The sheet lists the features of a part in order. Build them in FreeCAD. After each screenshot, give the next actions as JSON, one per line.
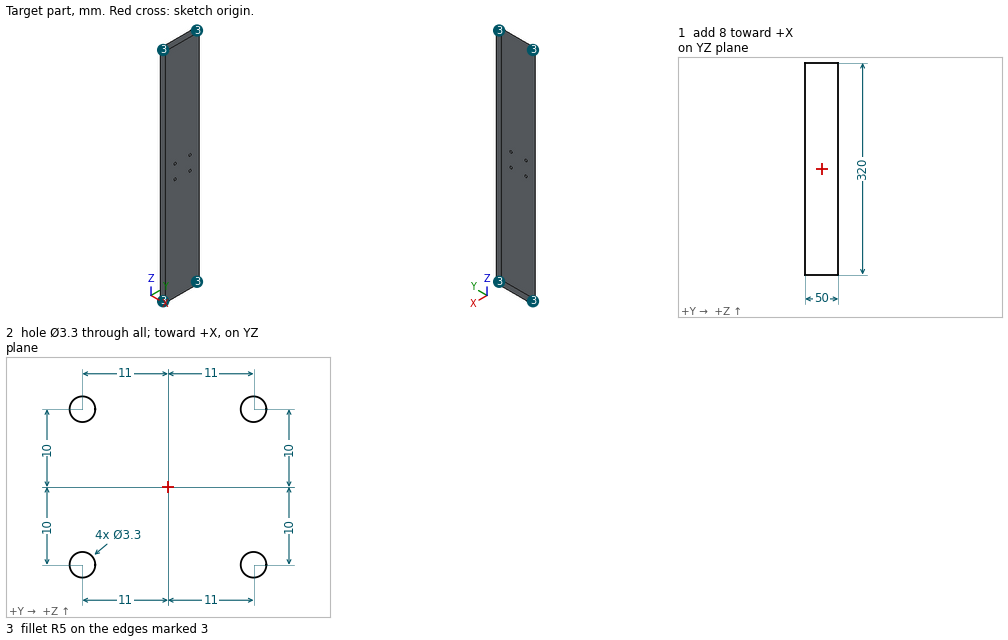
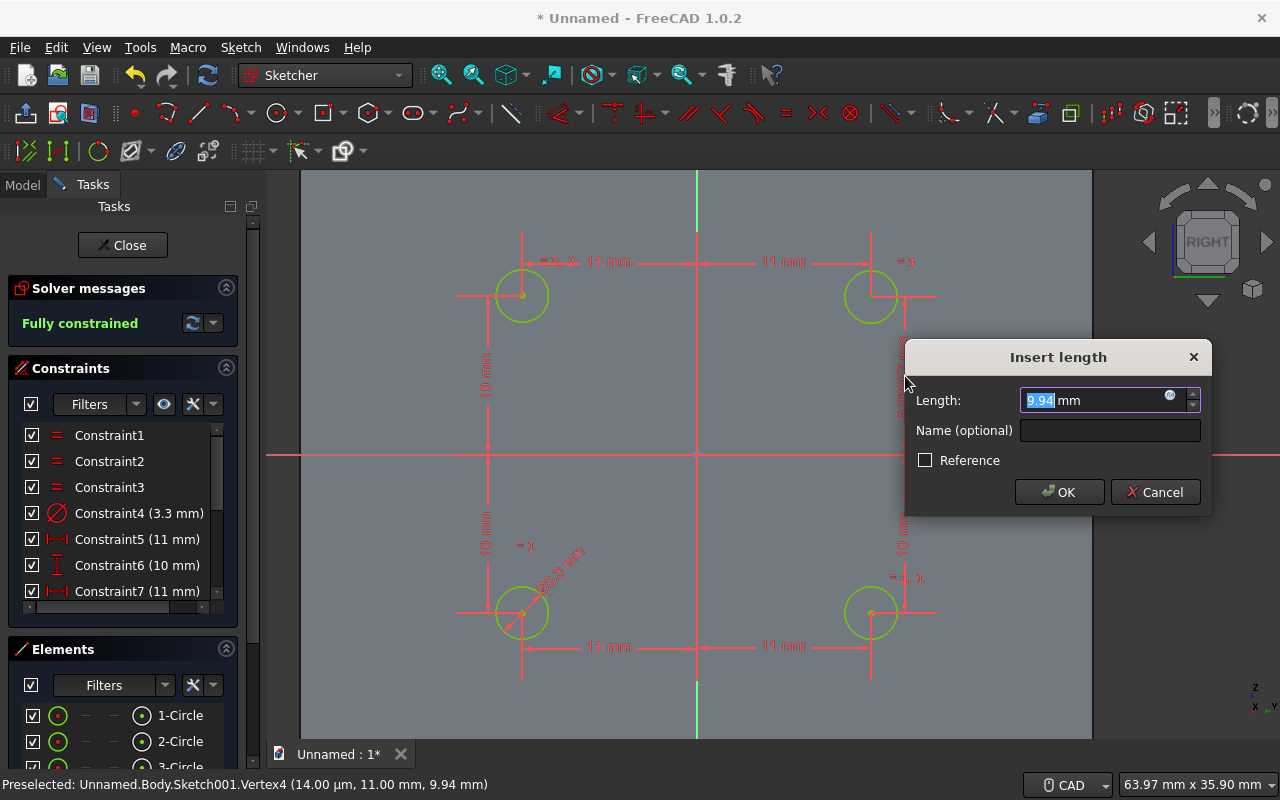
{"action": "type", "text": "10"}
{"action": "key", "text": "Return"}
{"action": "key", "text": "Escape"}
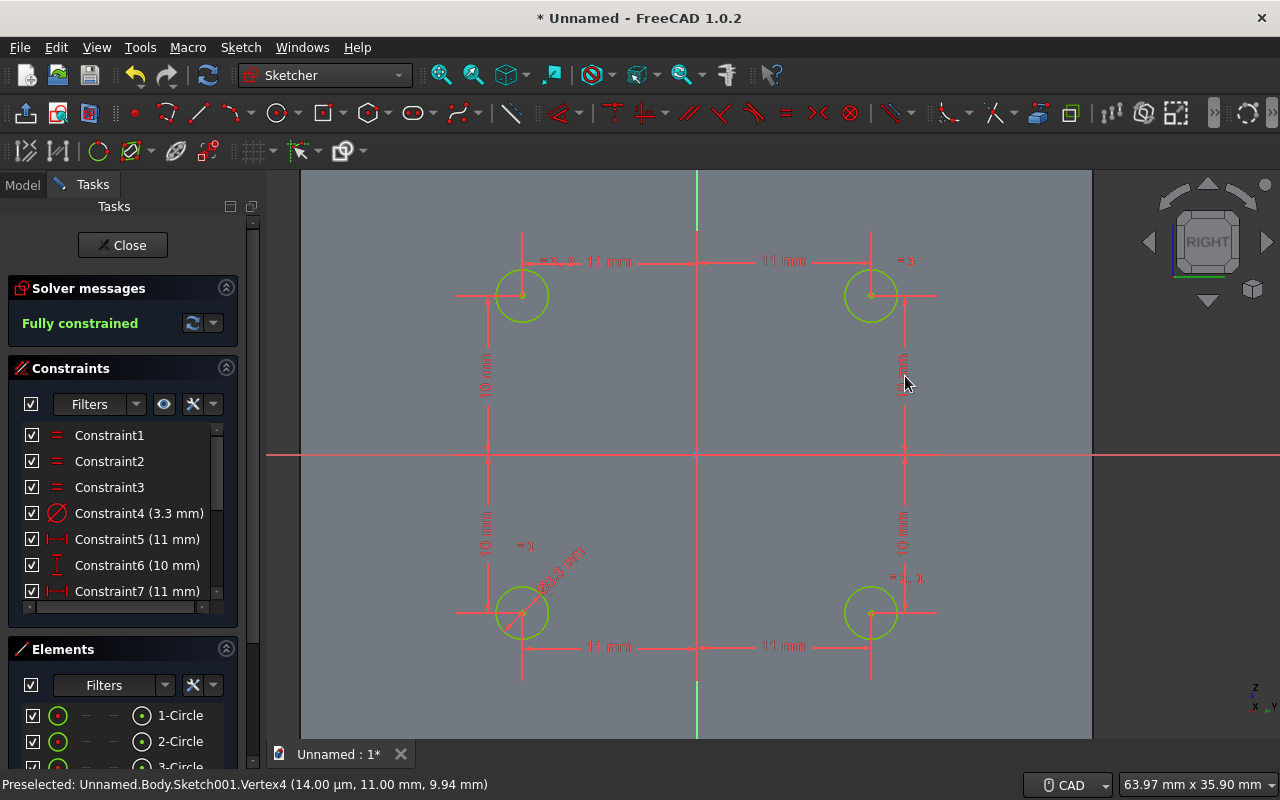
{"action": "left_click", "coordinate": [123, 245]}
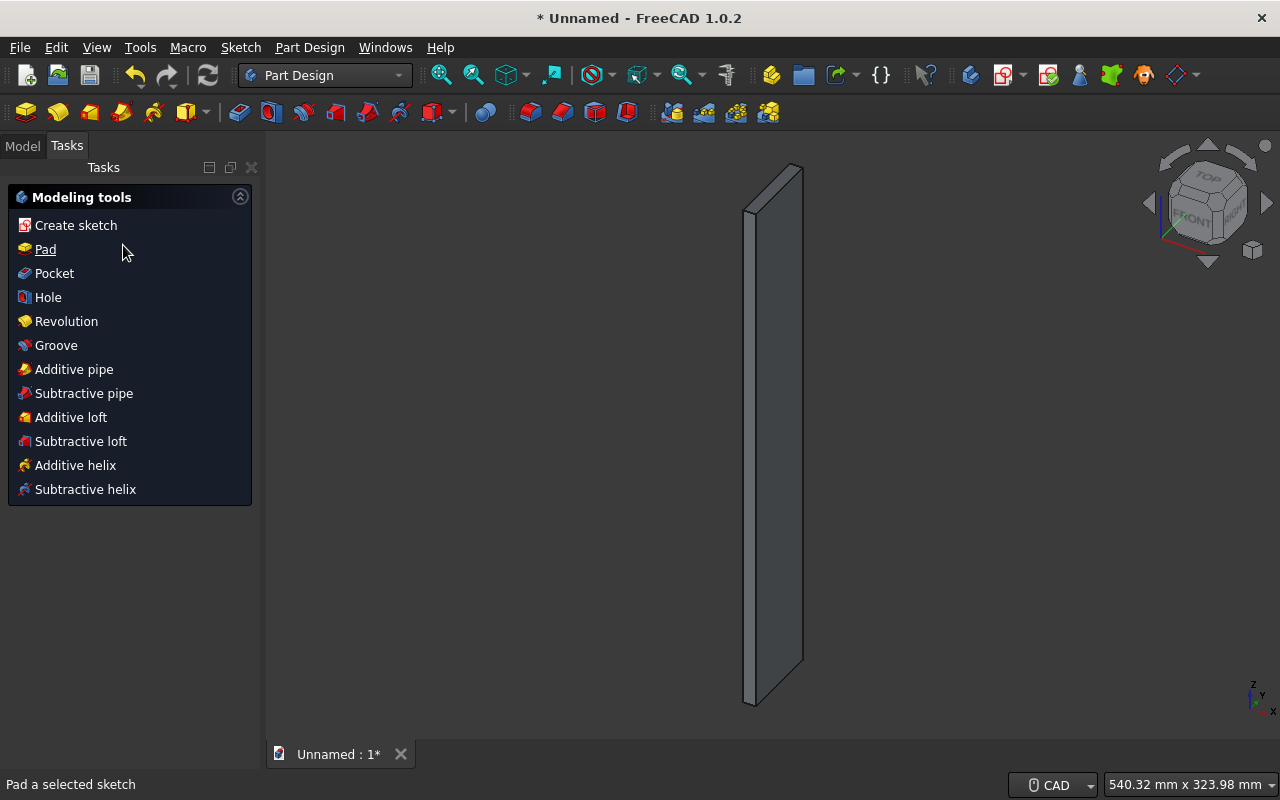
{"action": "left_click", "coordinate": [272, 112]}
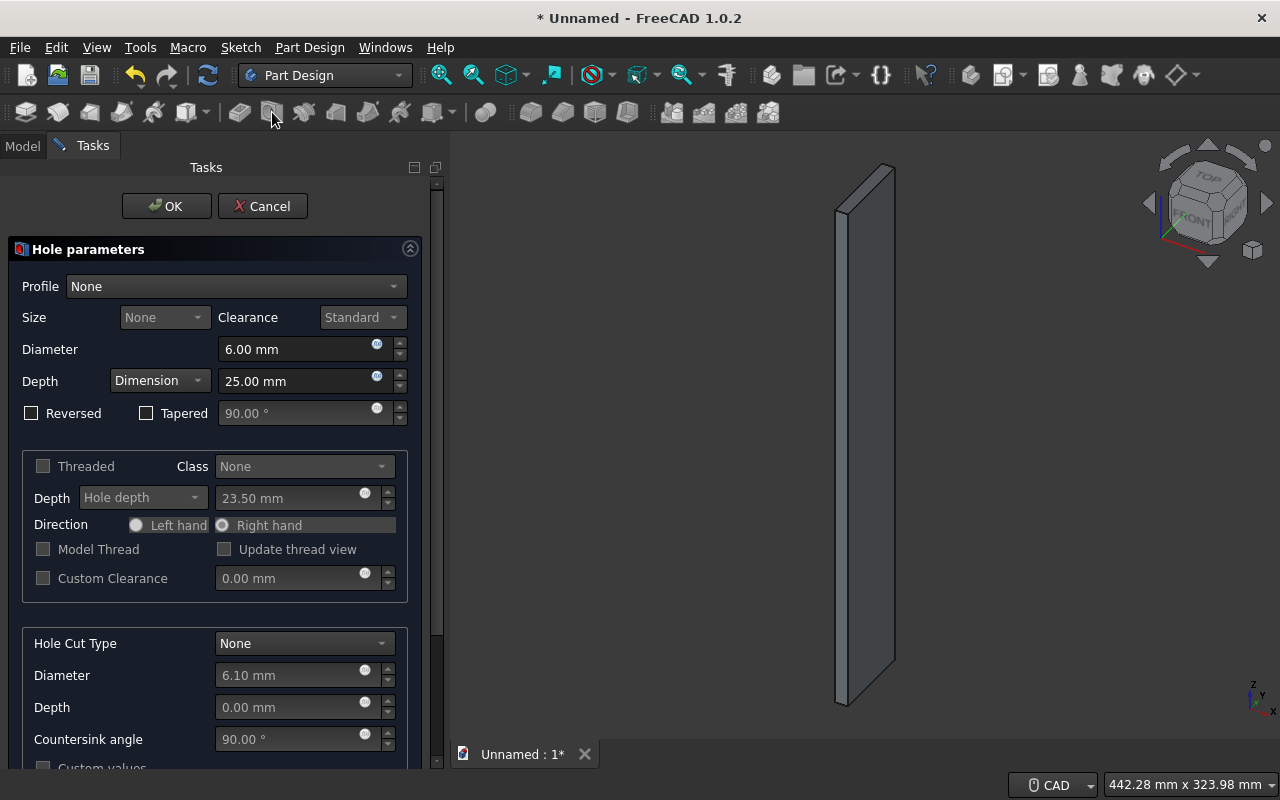
{"action": "triple_click", "coordinate": [305, 349]}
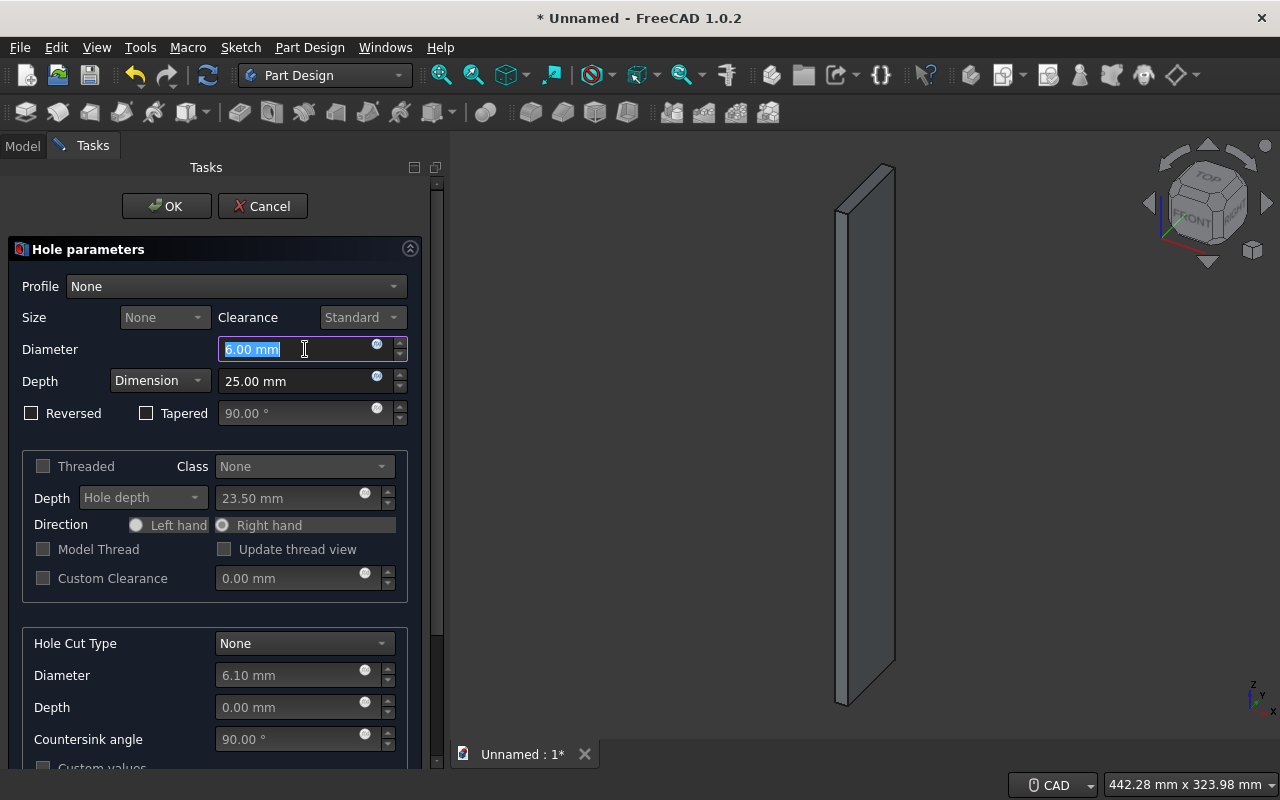
{"action": "type", "text": "3.3"}
{"action": "key", "text": "Tab"}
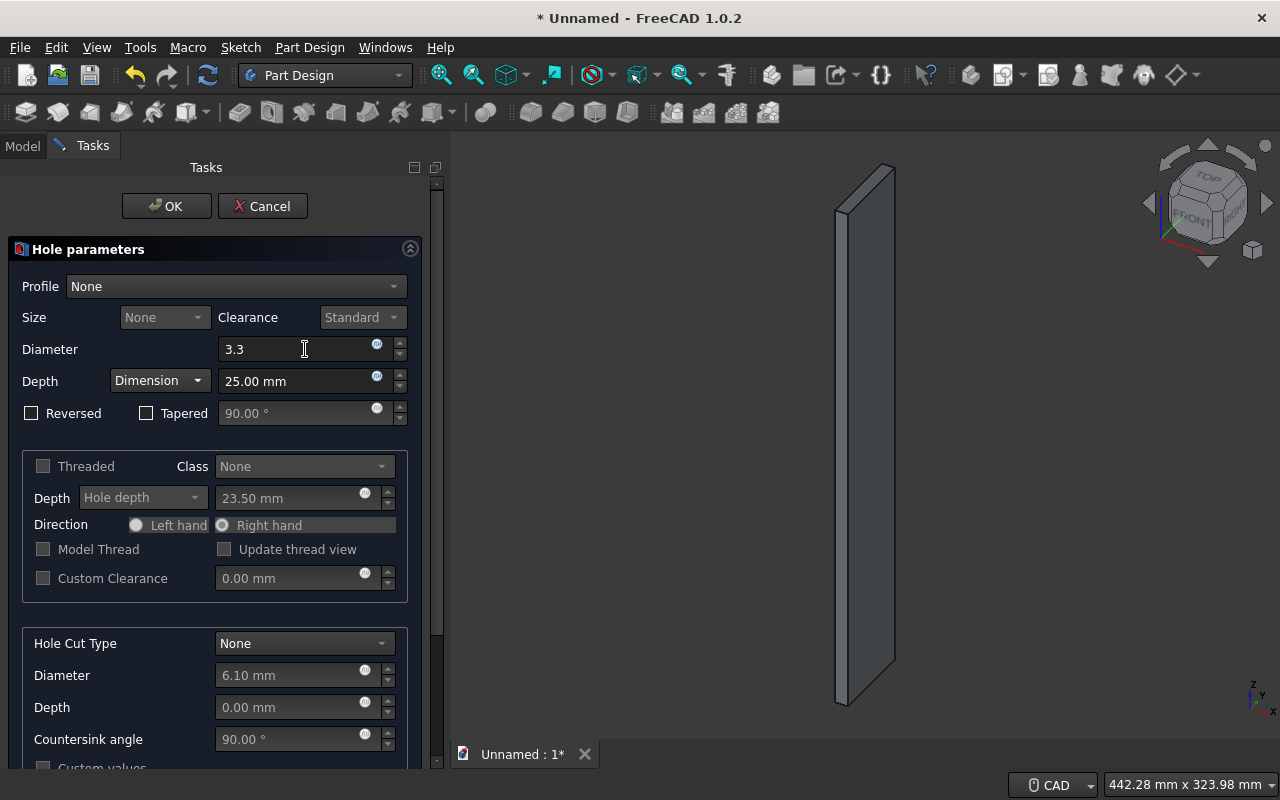
{"action": "left_click", "coordinate": [161, 380]}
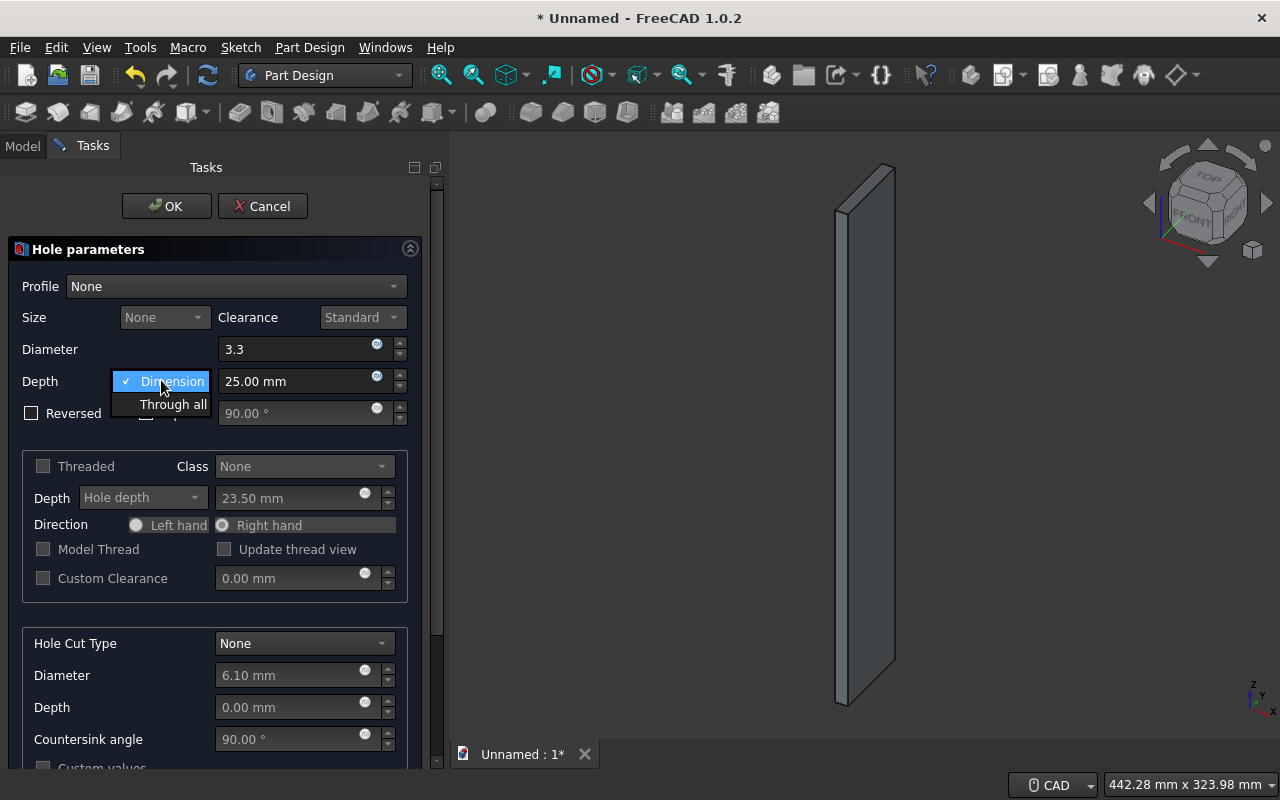
{"action": "left_click", "coordinate": [160, 404]}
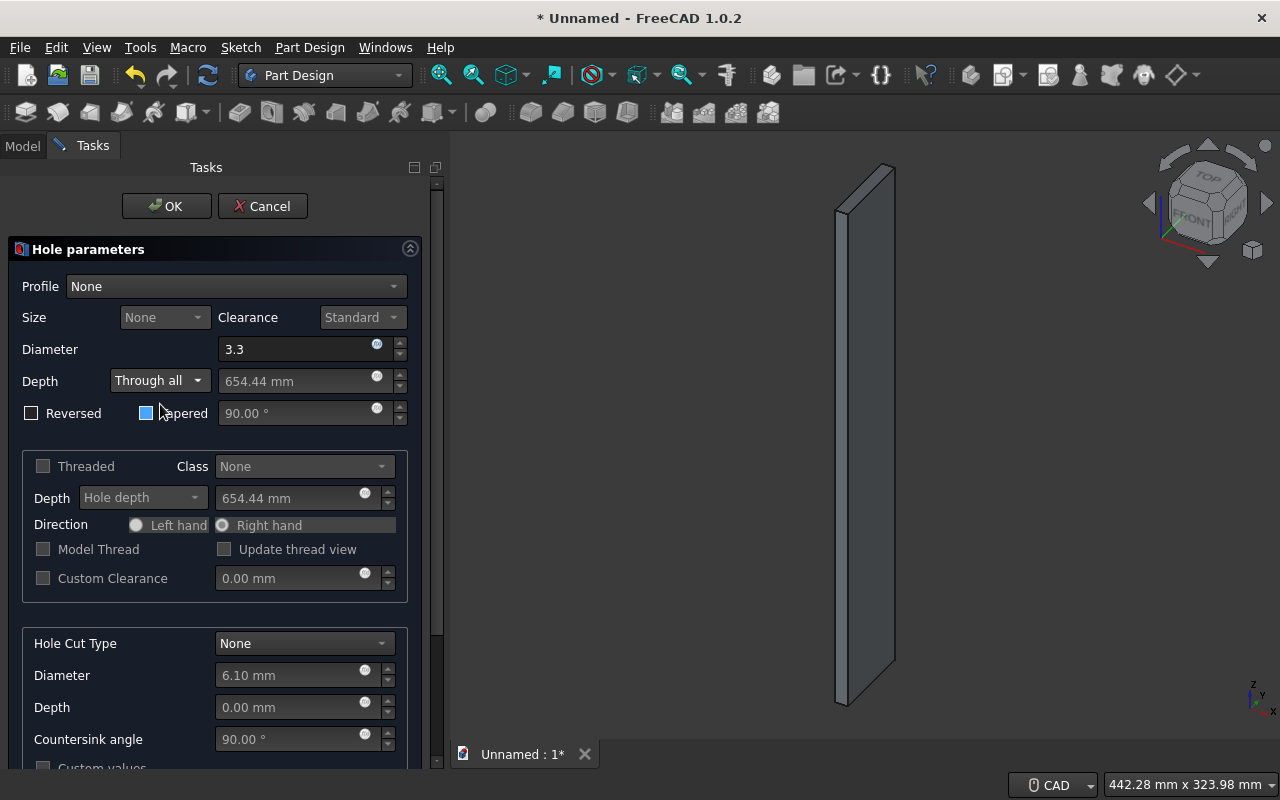
{"action": "left_click", "coordinate": [30, 413]}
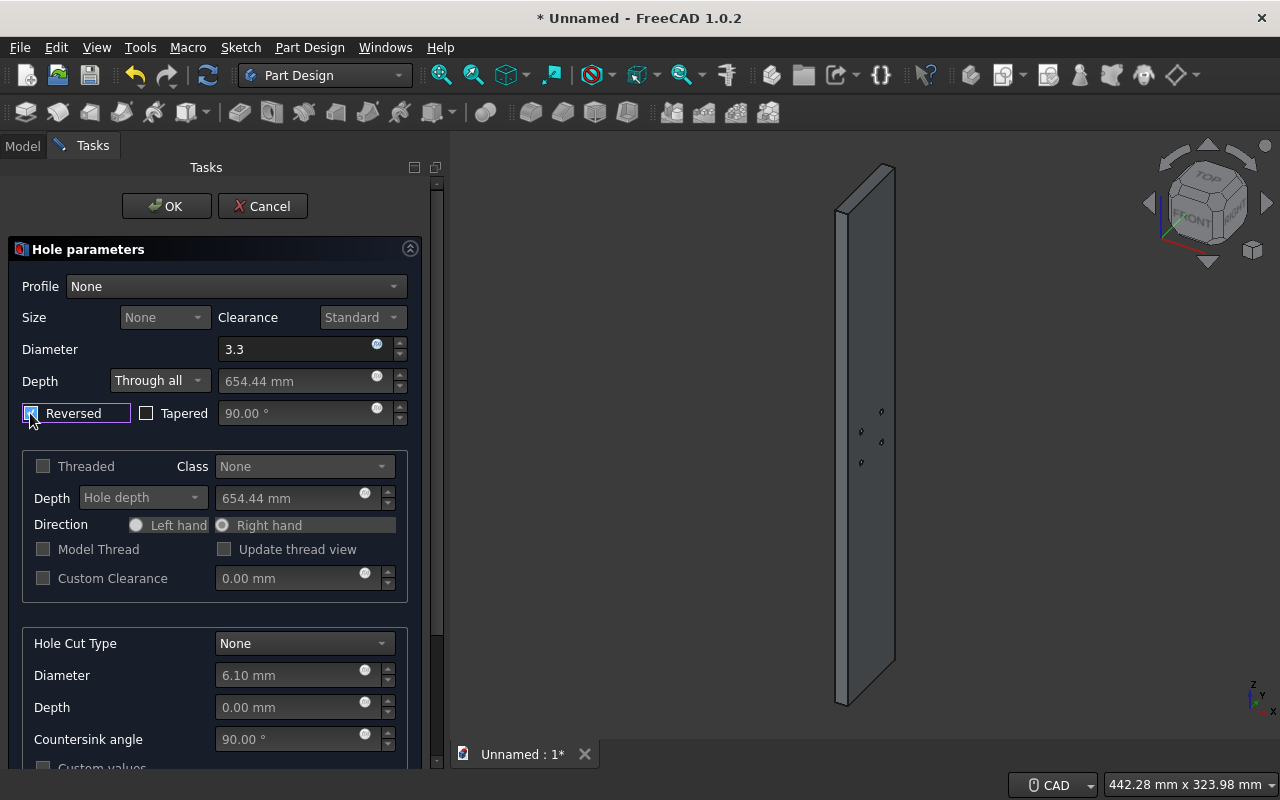
{"action": "left_click", "coordinate": [167, 206]}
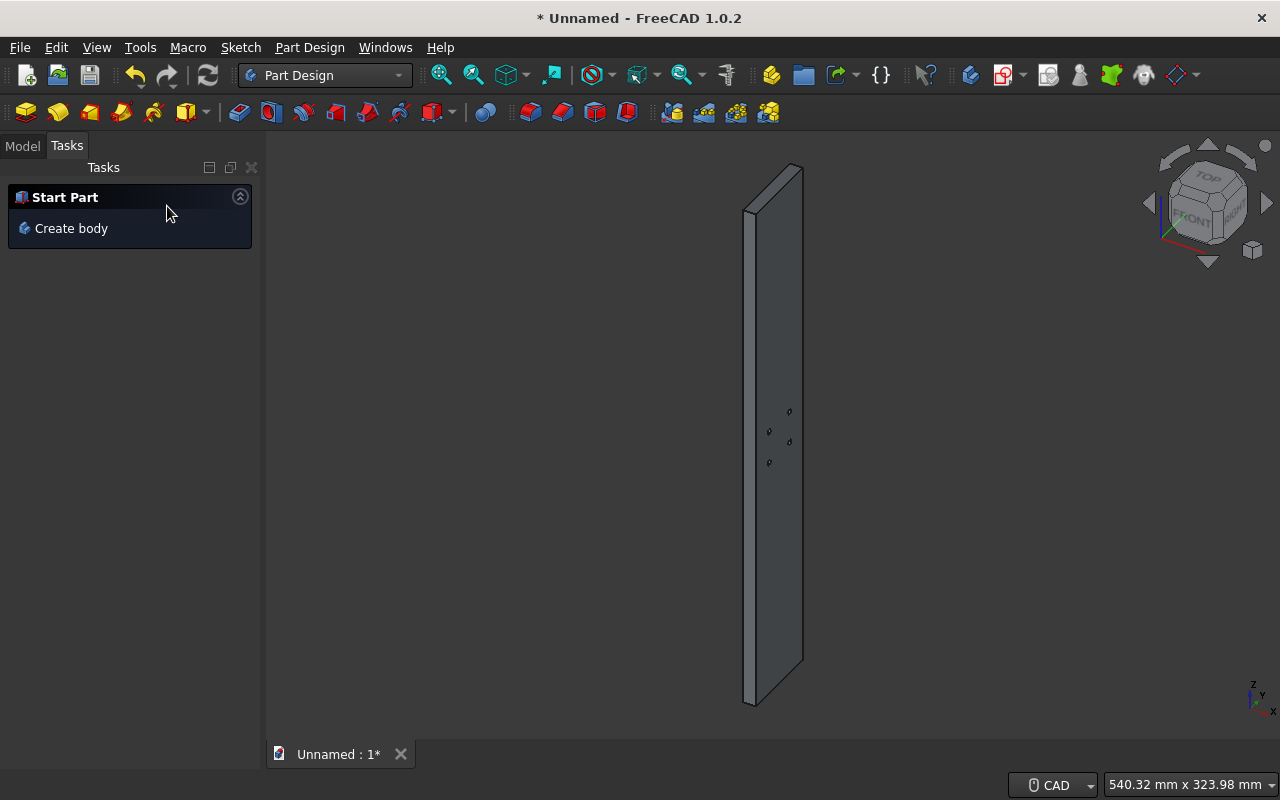
{"action": "left_click", "coordinate": [750, 211]}